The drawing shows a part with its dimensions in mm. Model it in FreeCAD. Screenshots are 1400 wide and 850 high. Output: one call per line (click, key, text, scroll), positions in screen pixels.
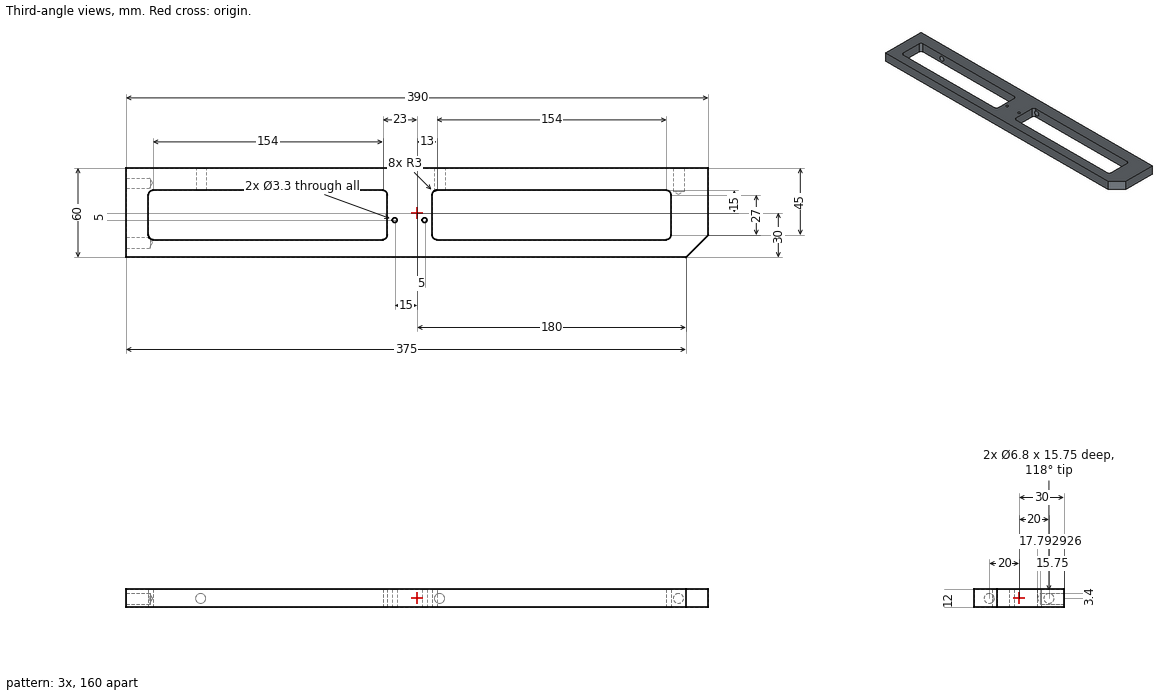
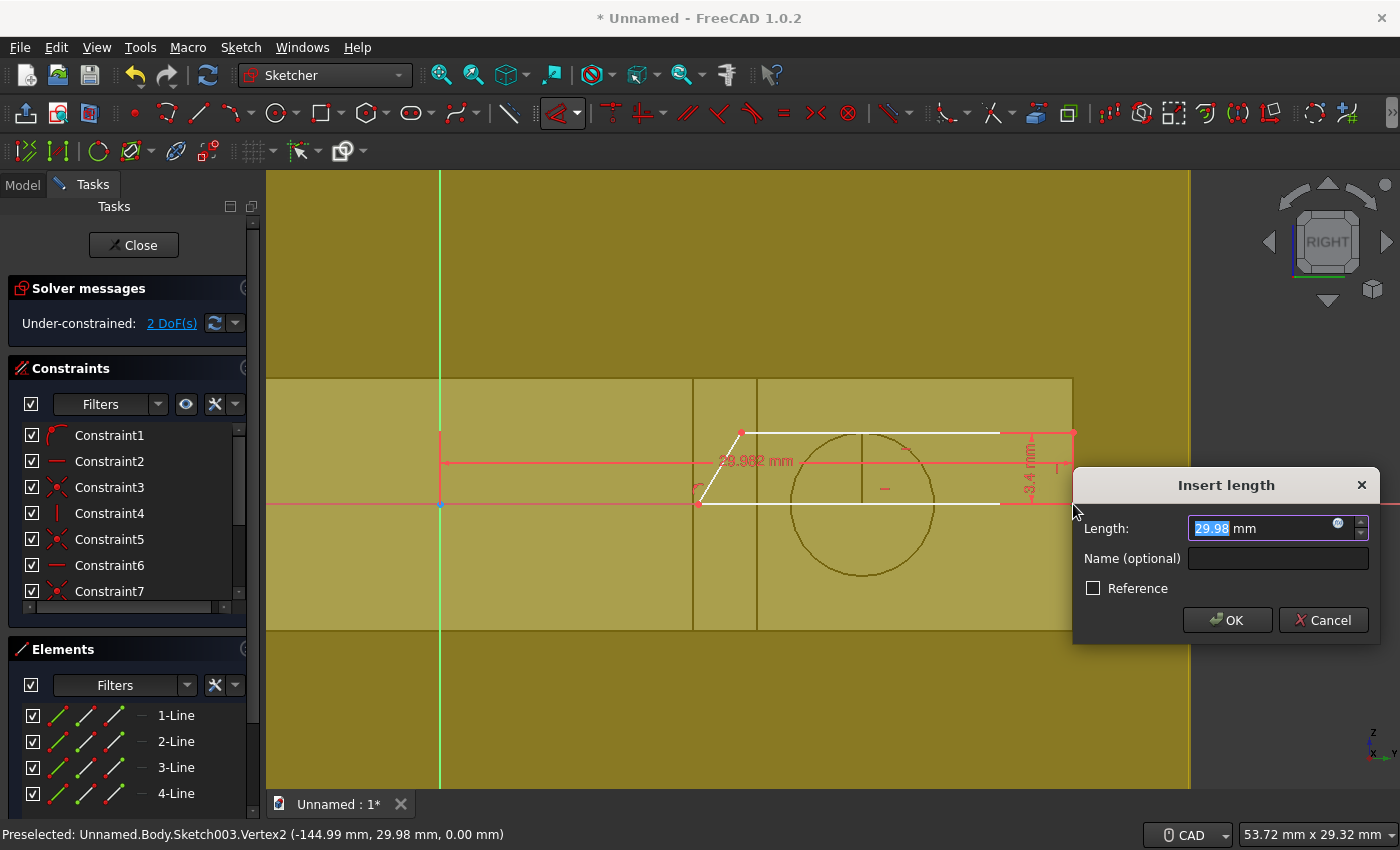
text(30)
key(Return)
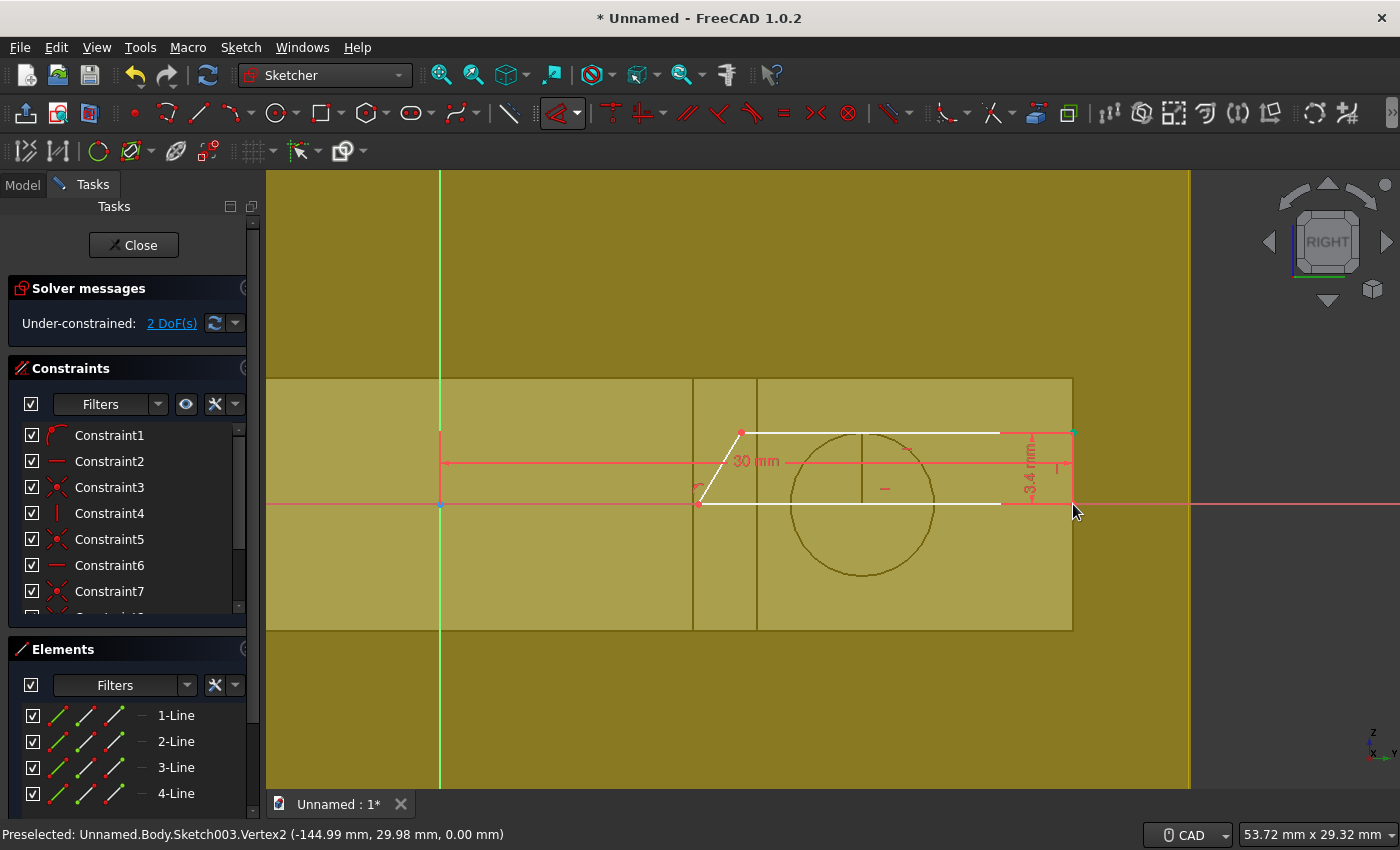
click(974, 433)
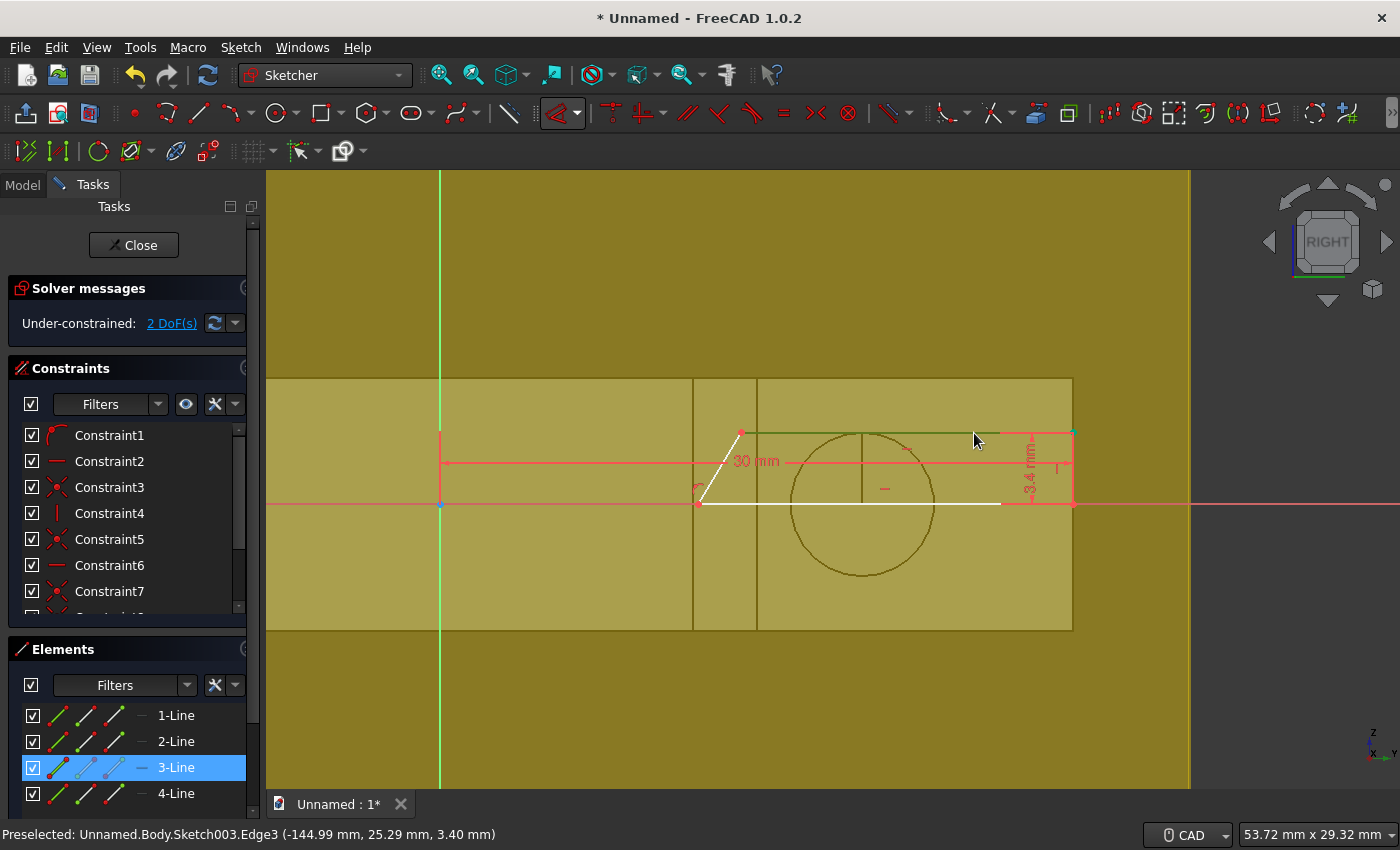
click(580, 114)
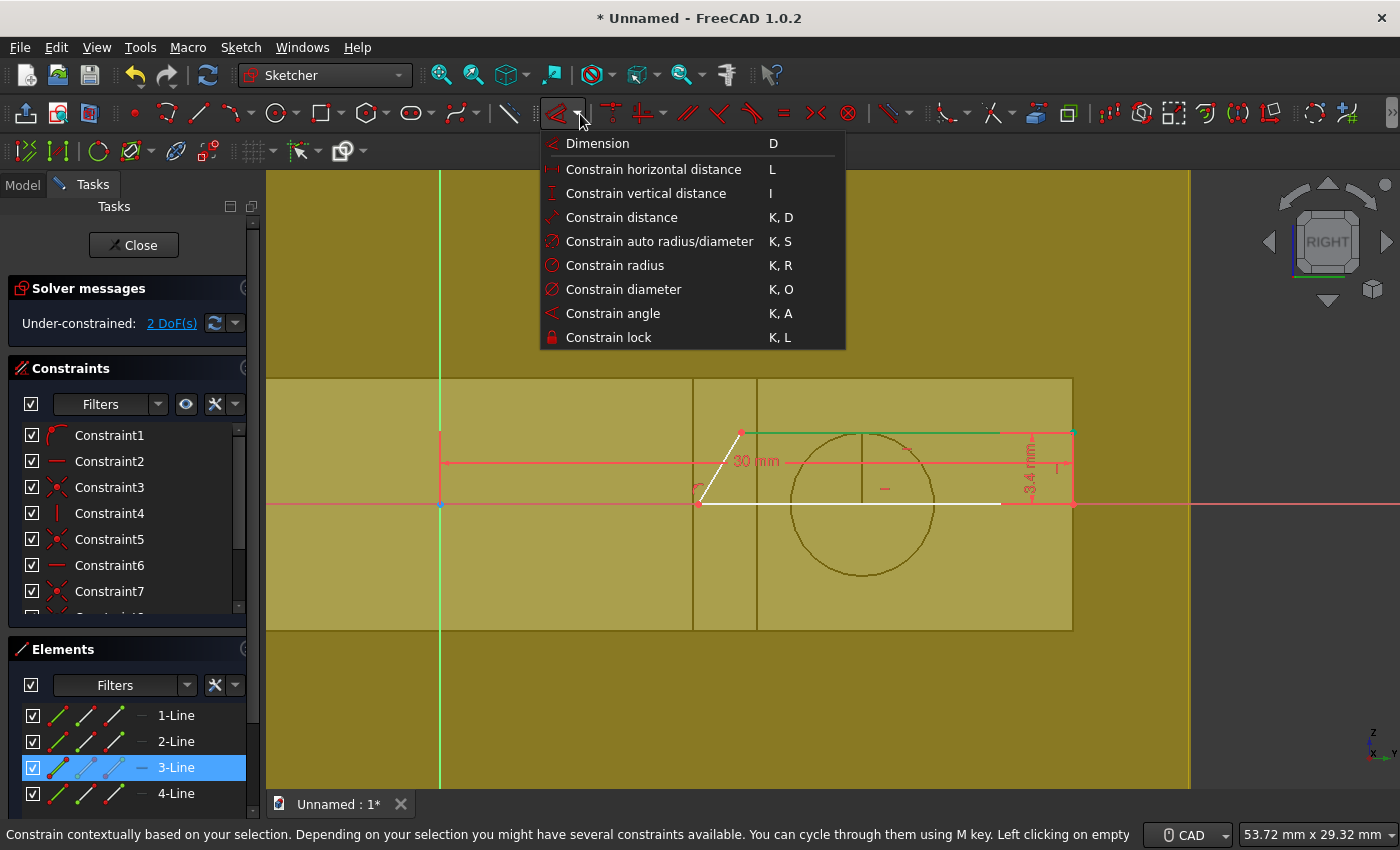
click(693, 169)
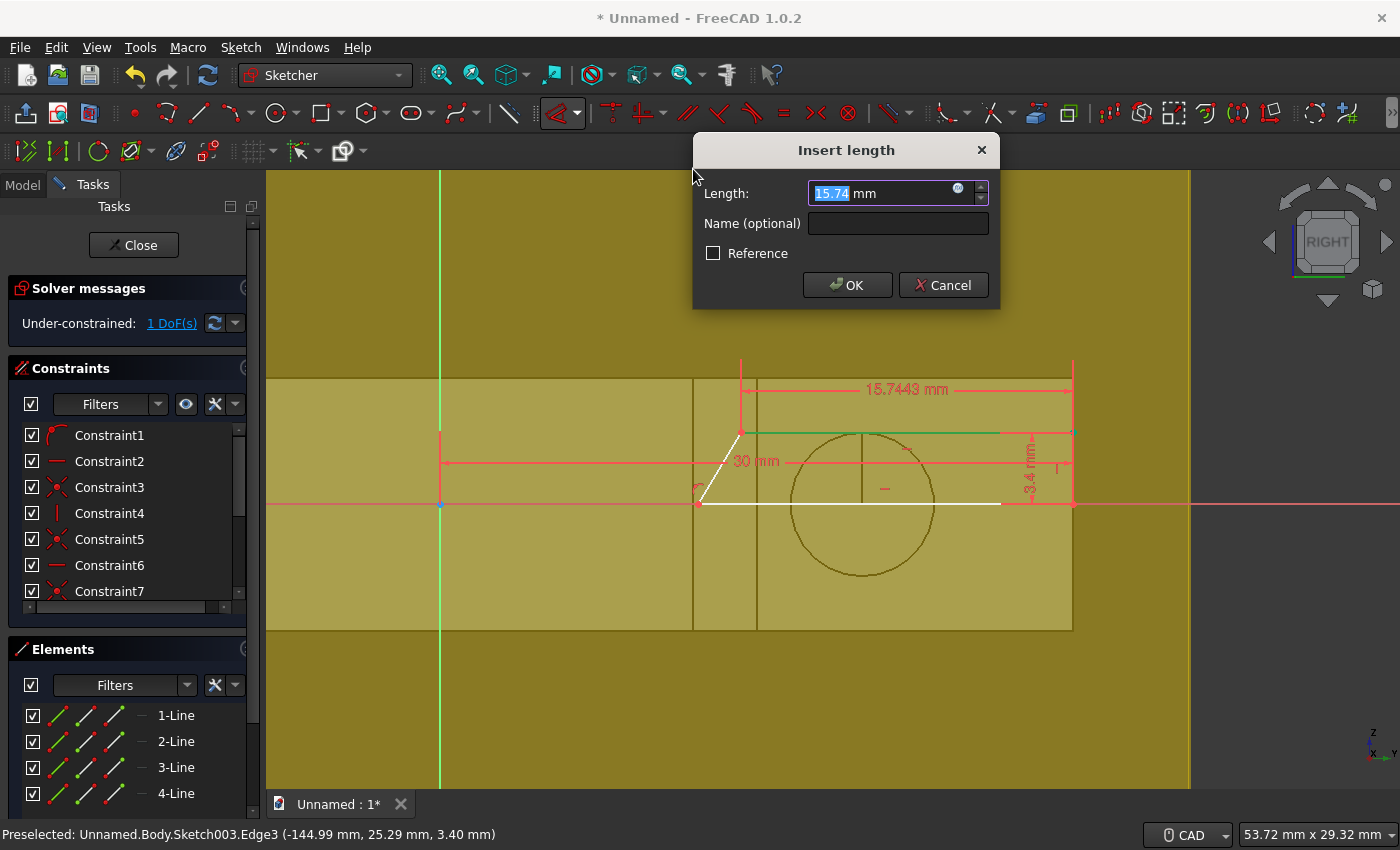
text(15.75)
key(Return)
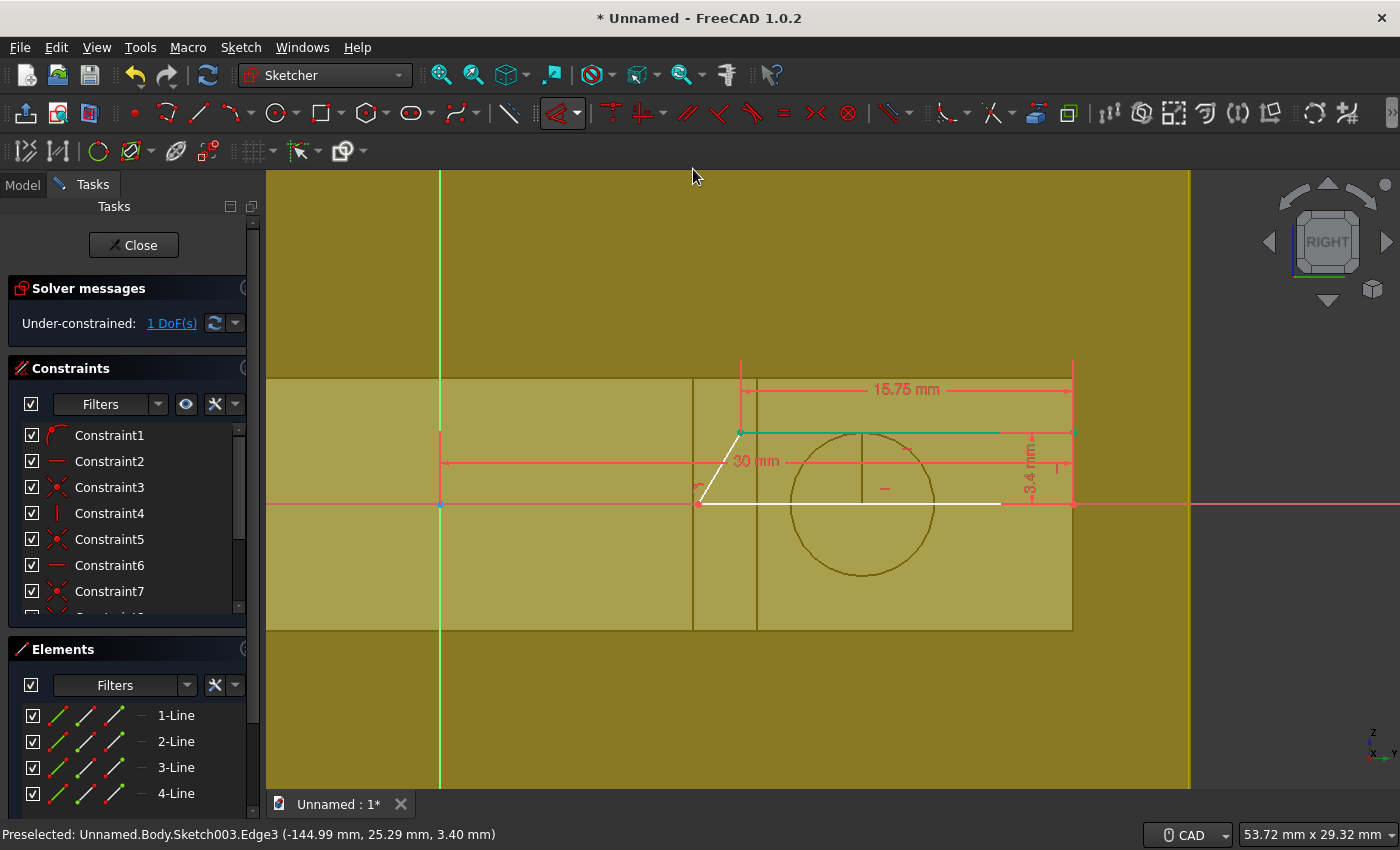
click(811, 504)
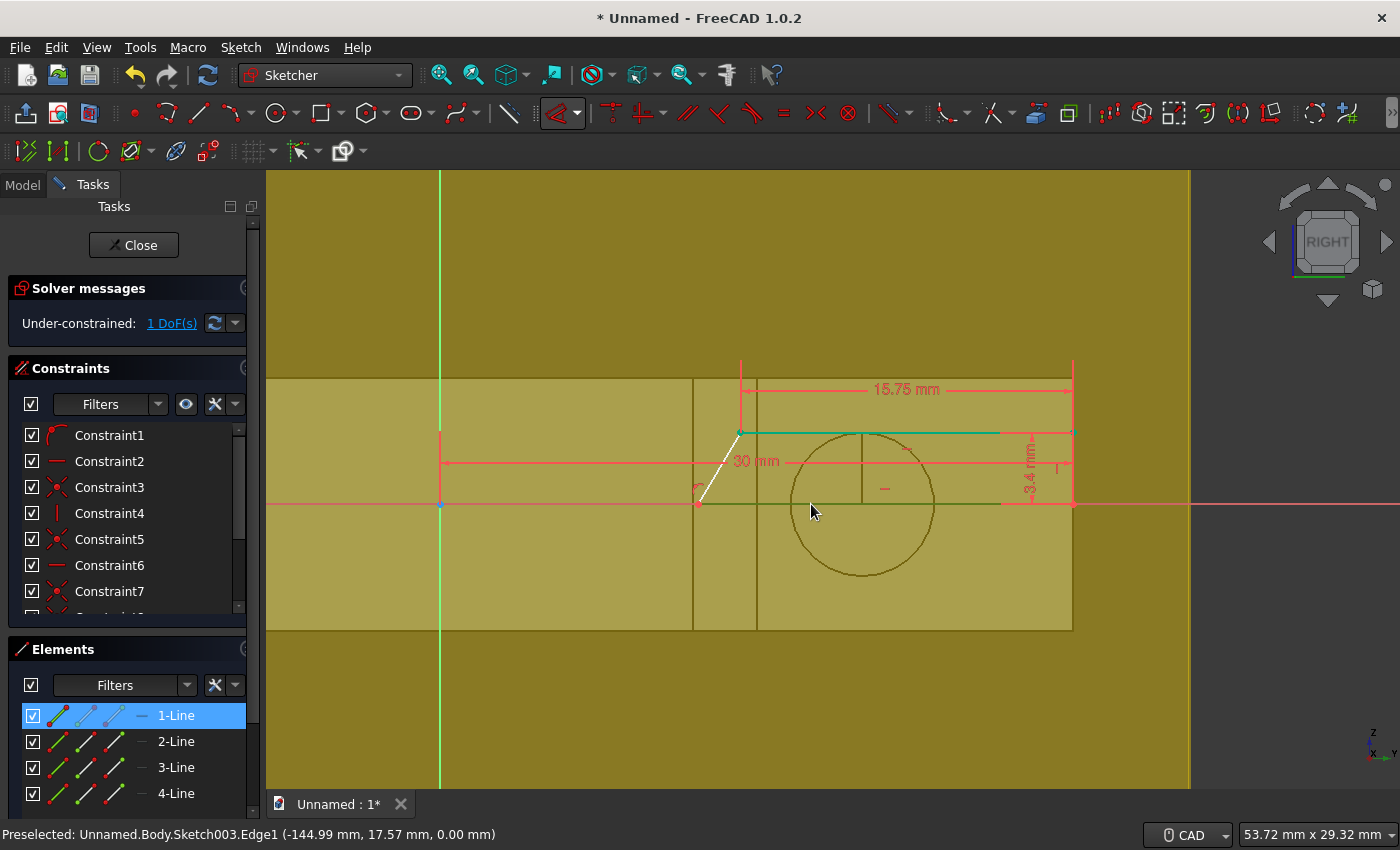
key(l)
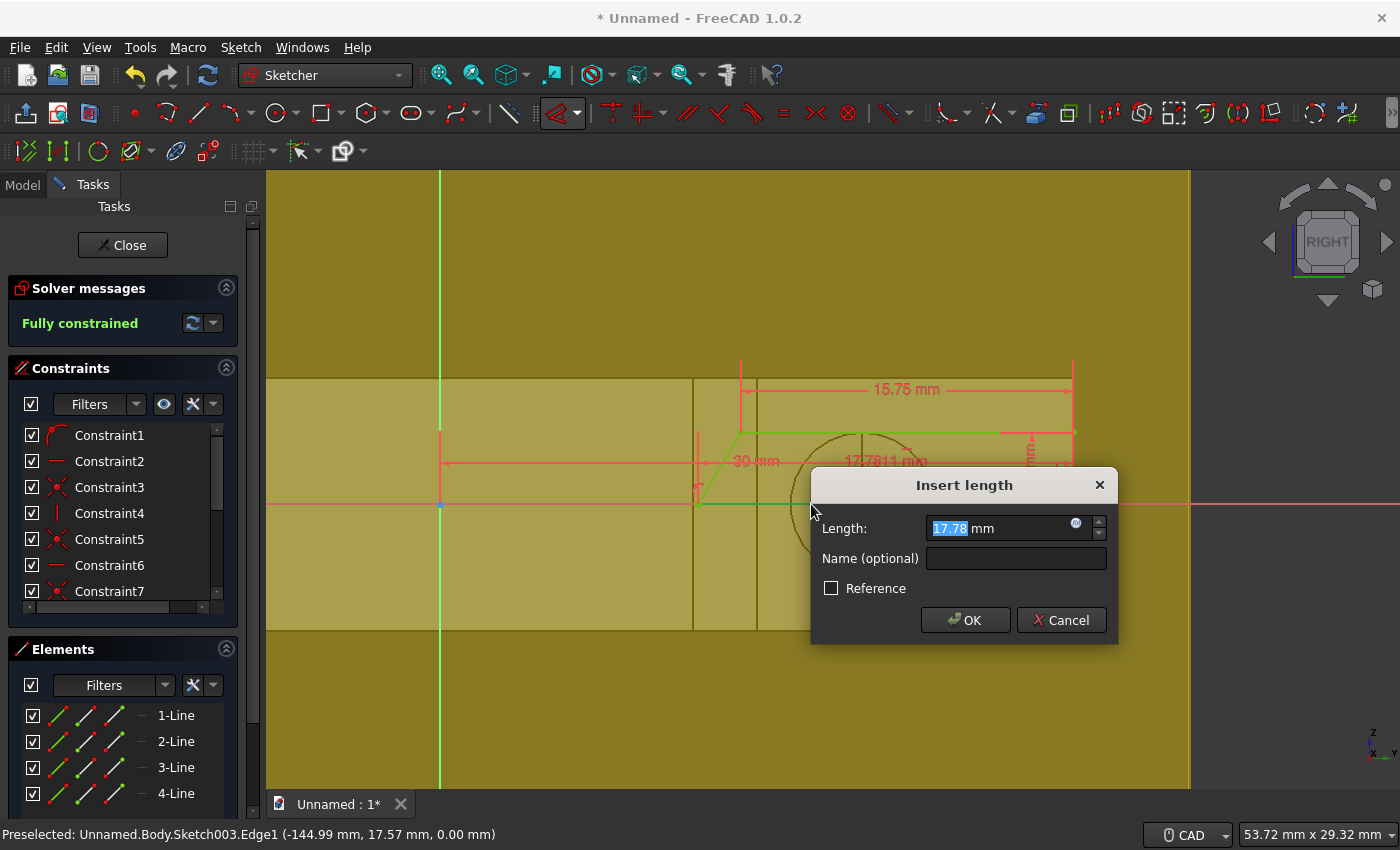
text(17.792926)
key(Return)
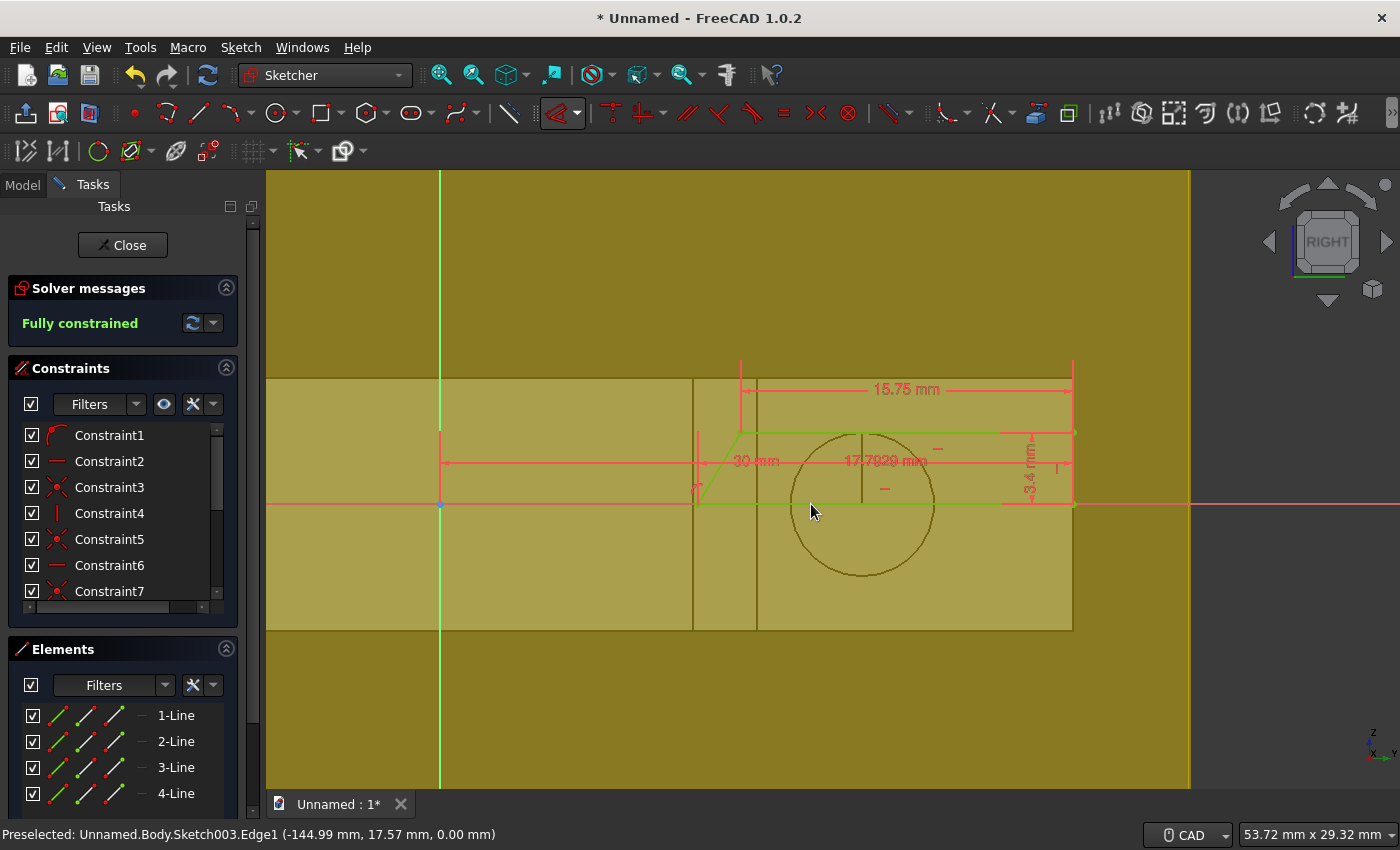
click(123, 245)